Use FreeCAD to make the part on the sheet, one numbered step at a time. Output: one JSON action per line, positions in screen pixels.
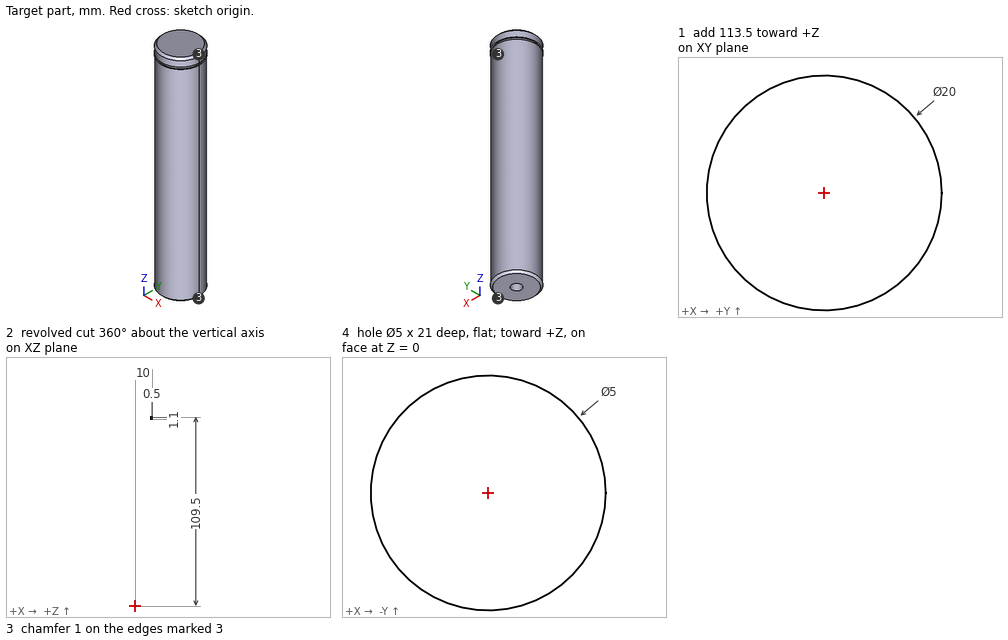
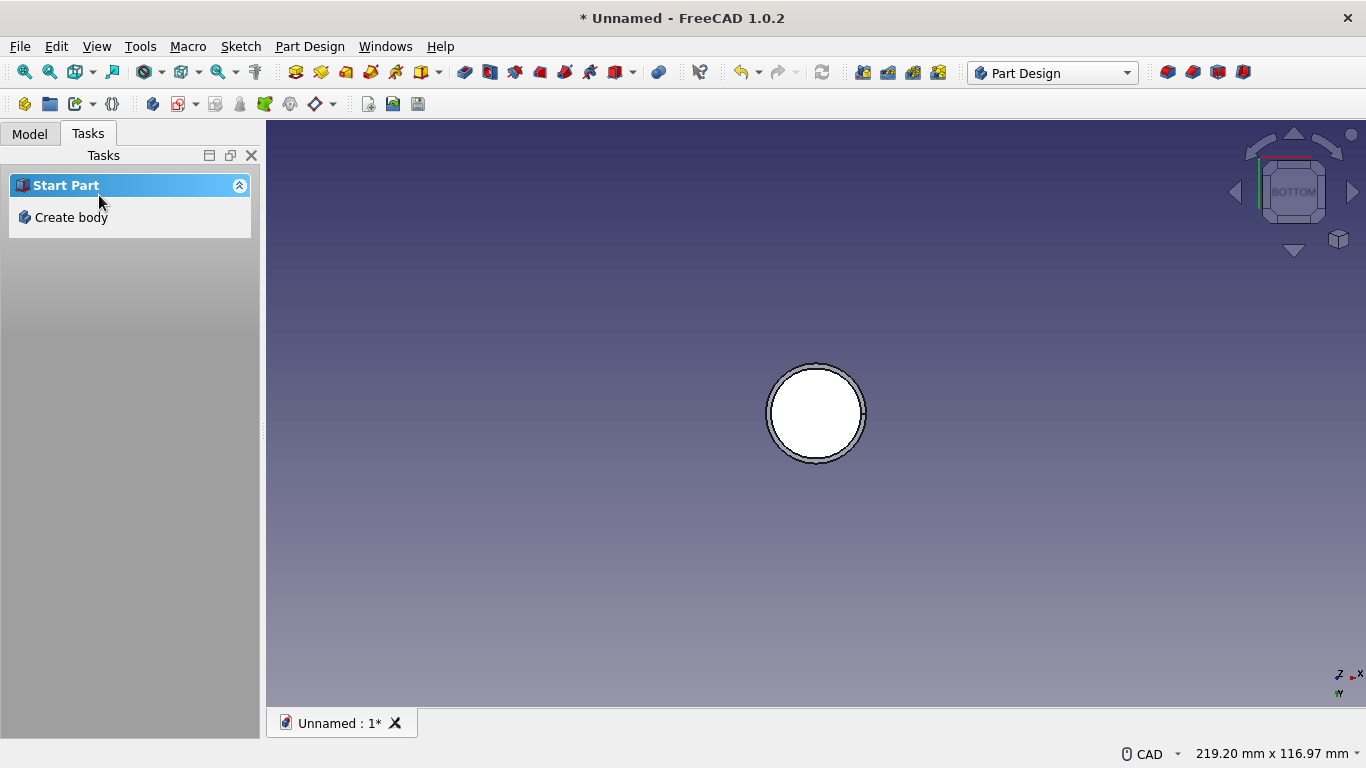
{"action": "left_click", "coordinate": [816, 412]}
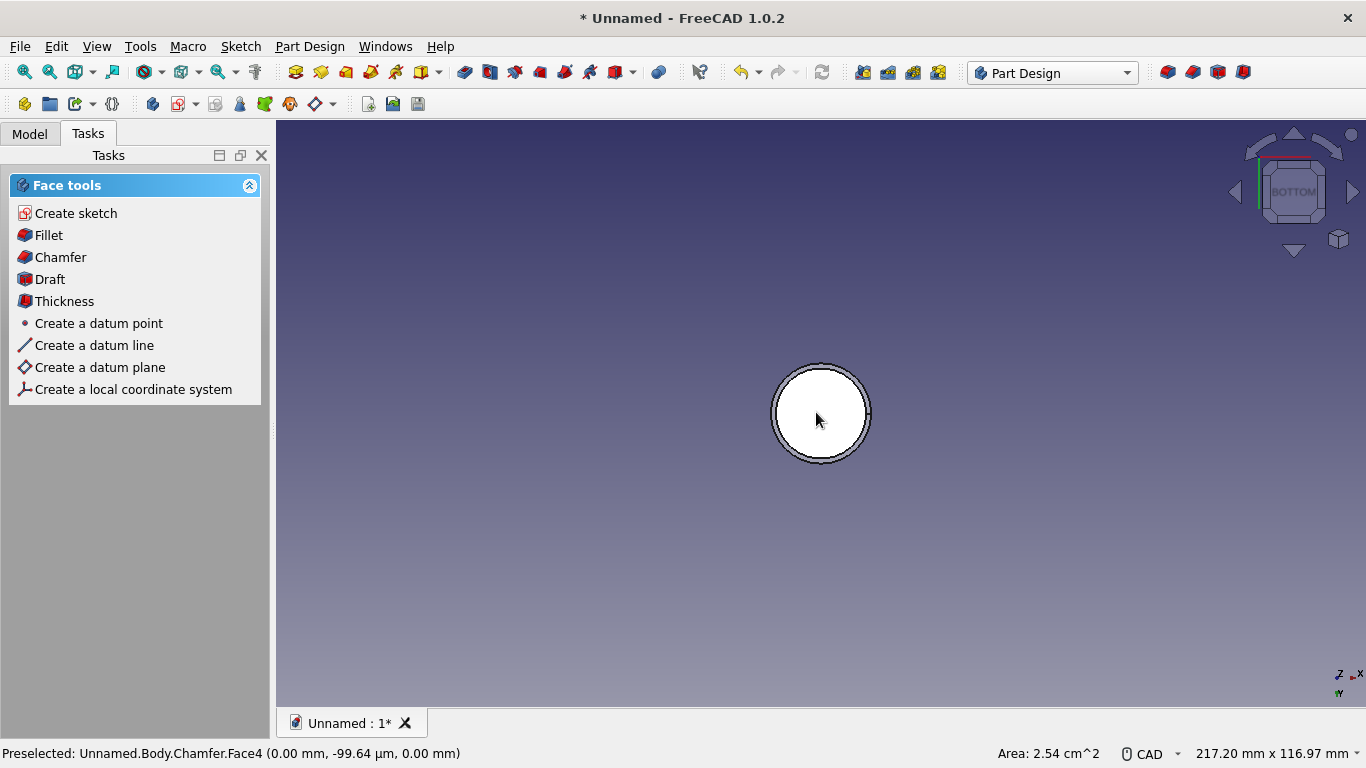
{"action": "left_click", "coordinate": [178, 104]}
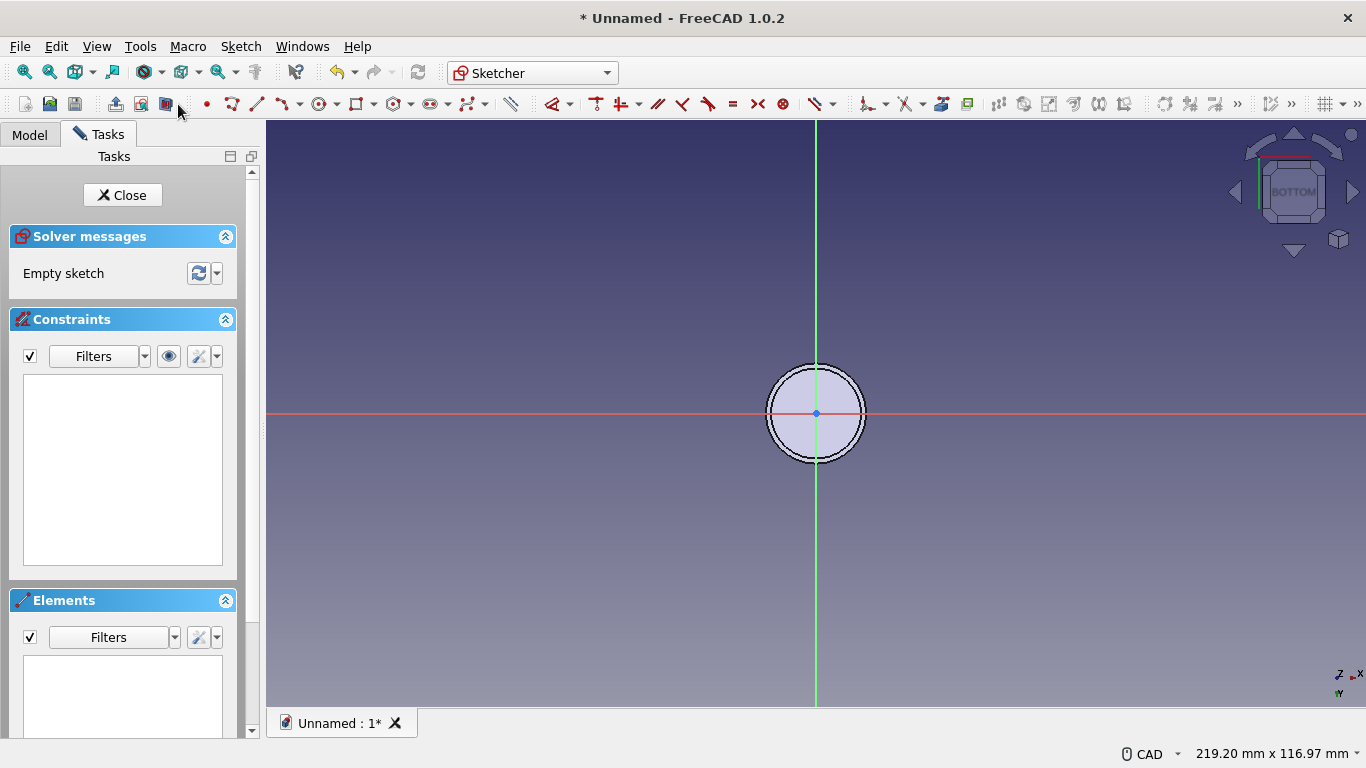
{"action": "scroll", "coordinate": [820, 414], "scroll_direction": "up", "scroll_amount": 14}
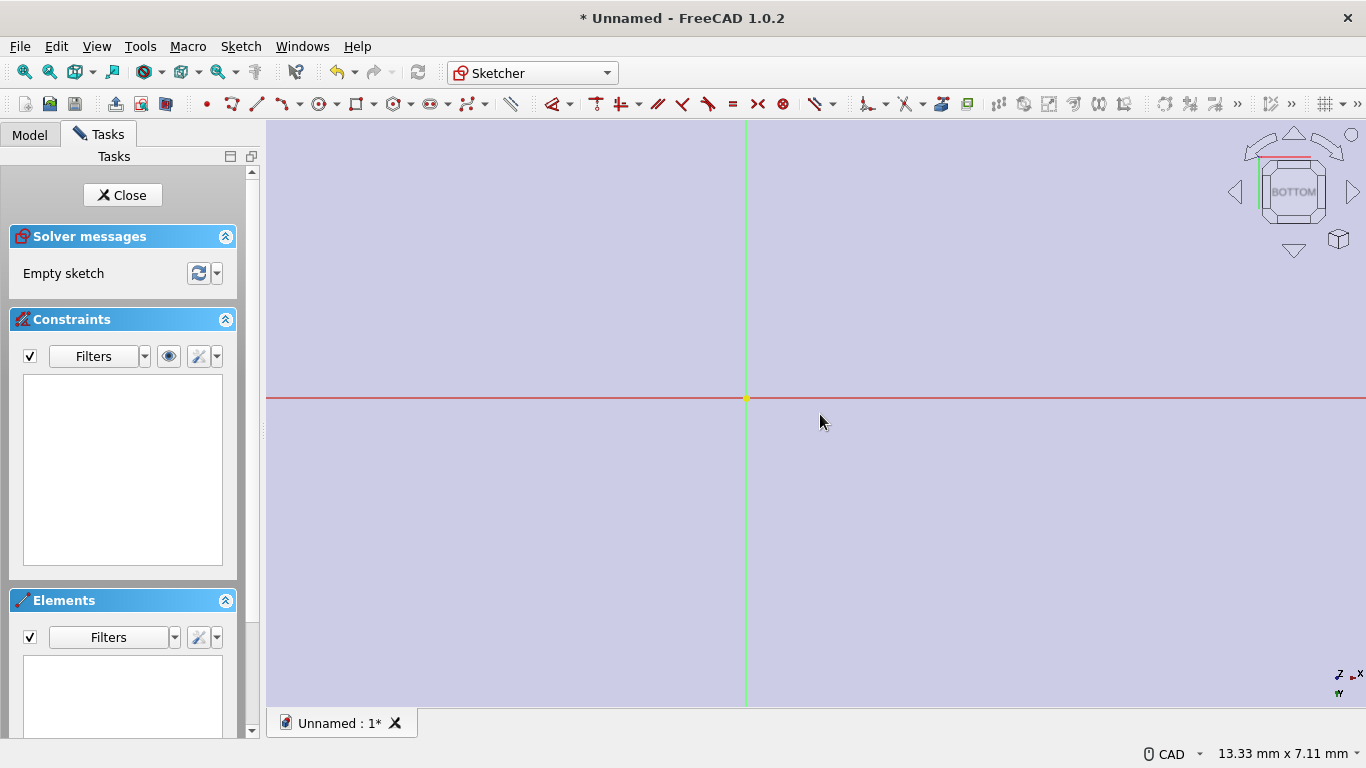
{"action": "left_click", "coordinate": [318, 104]}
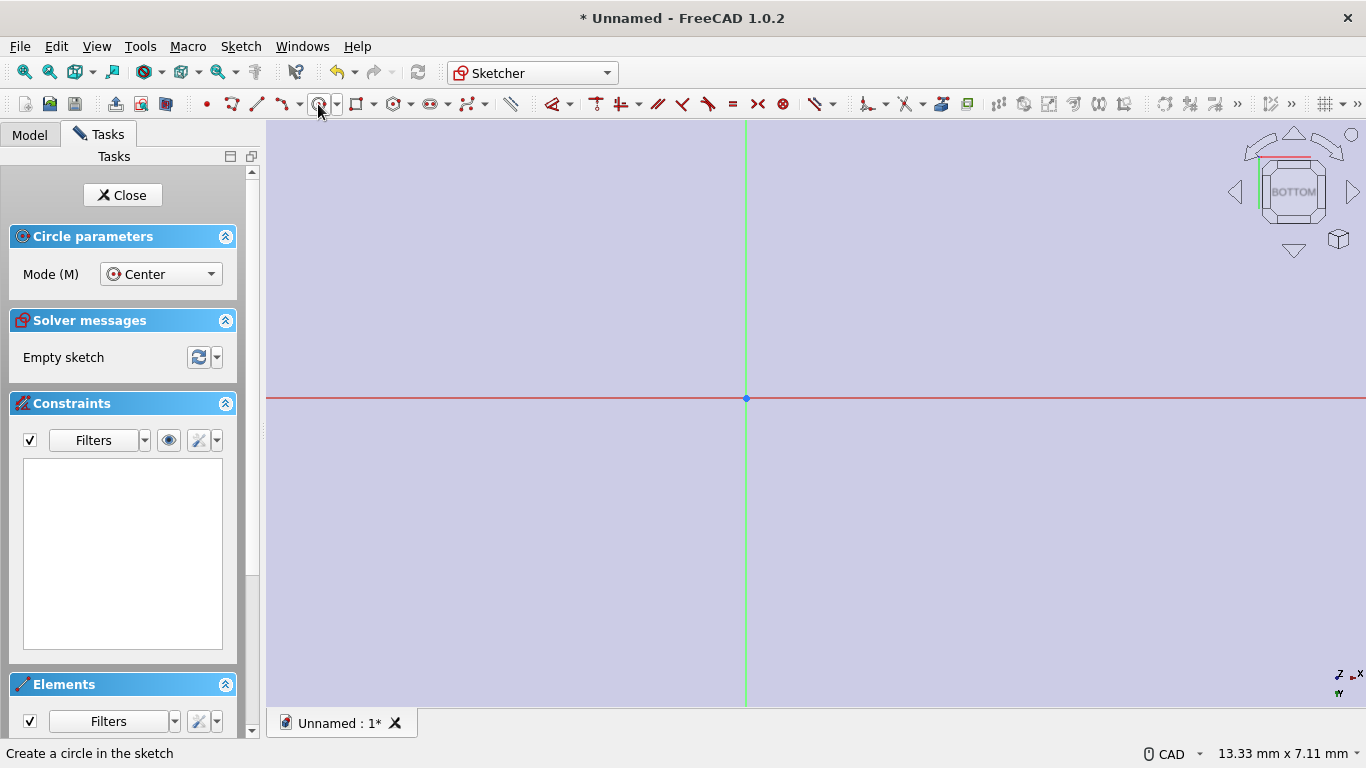
{"action": "left_click", "coordinate": [746, 398]}
{"action": "left_click", "coordinate": [892, 252]}
{"action": "key", "text": "Escape"}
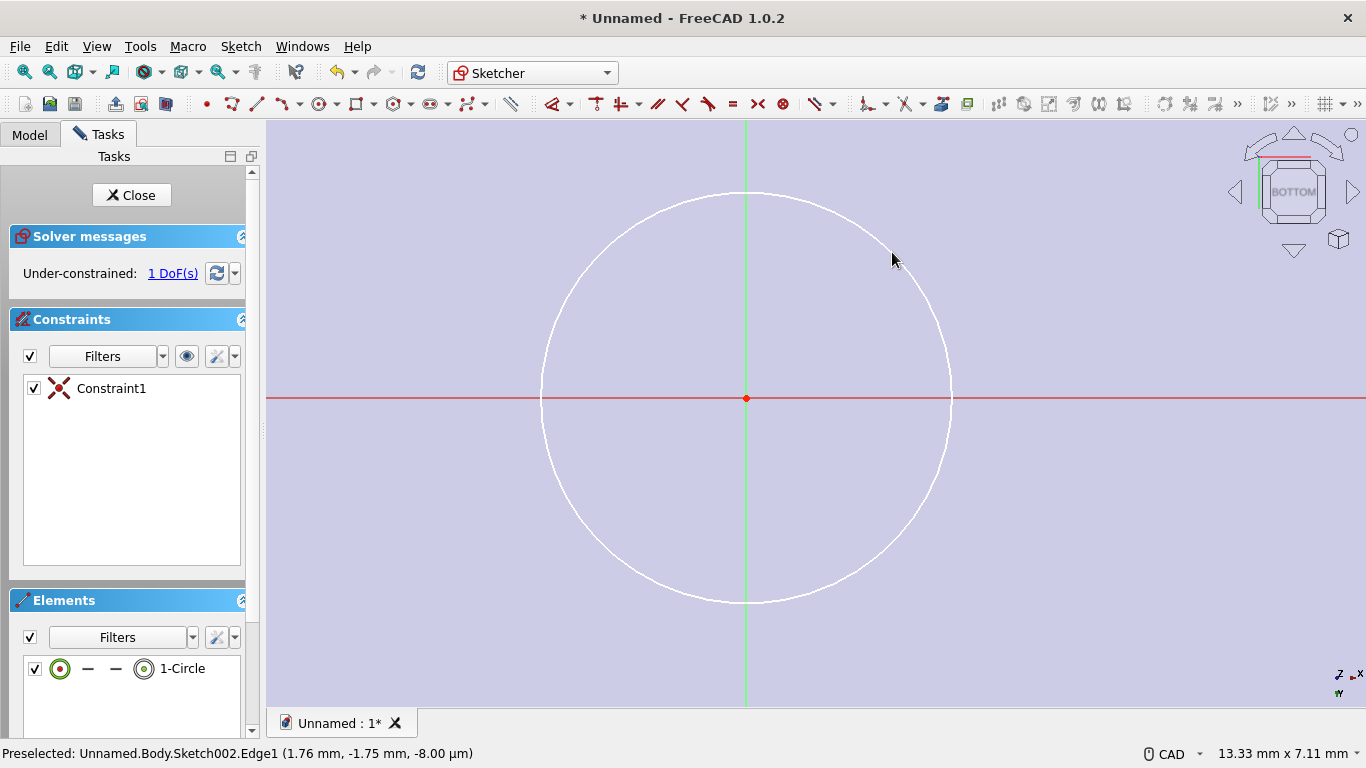
{"action": "key", "text": "d"}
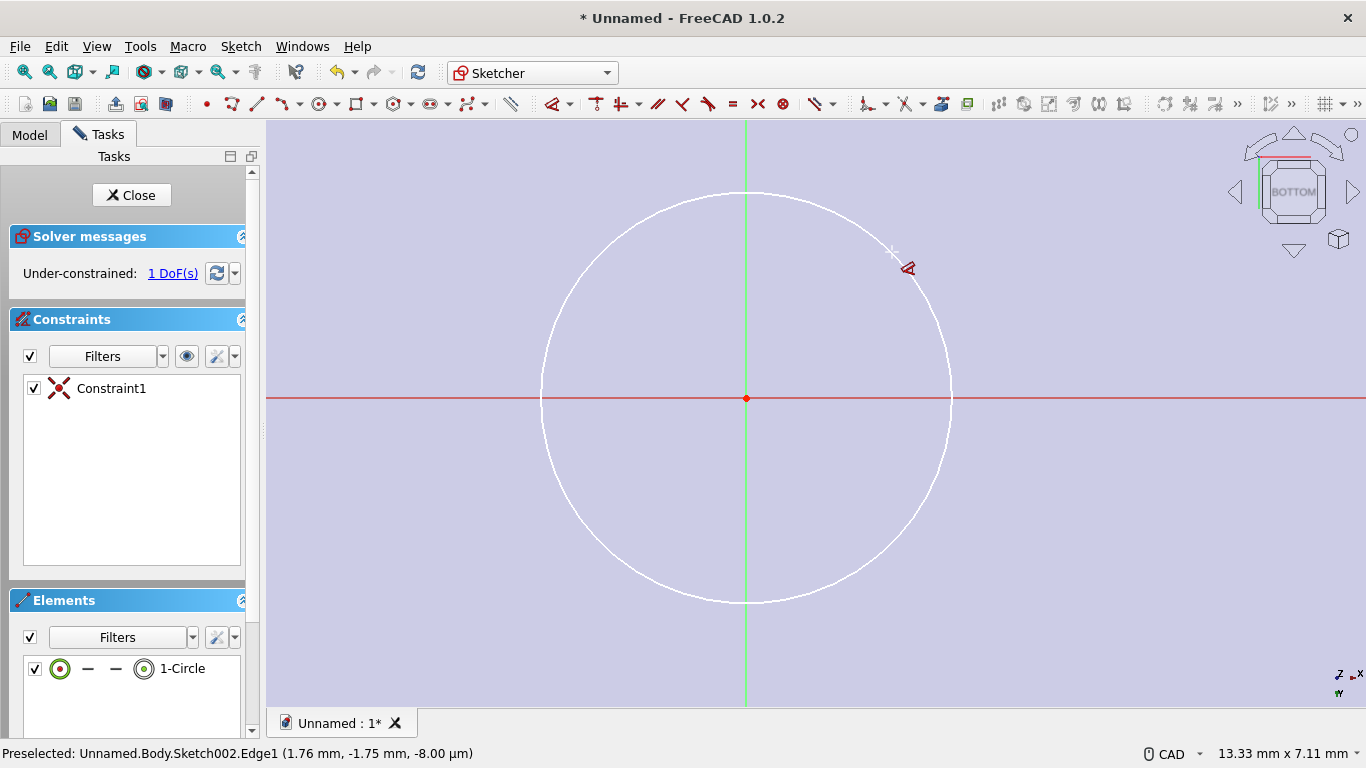
{"action": "left_click", "coordinate": [891, 252]}
{"action": "left_click", "coordinate": [914, 229]}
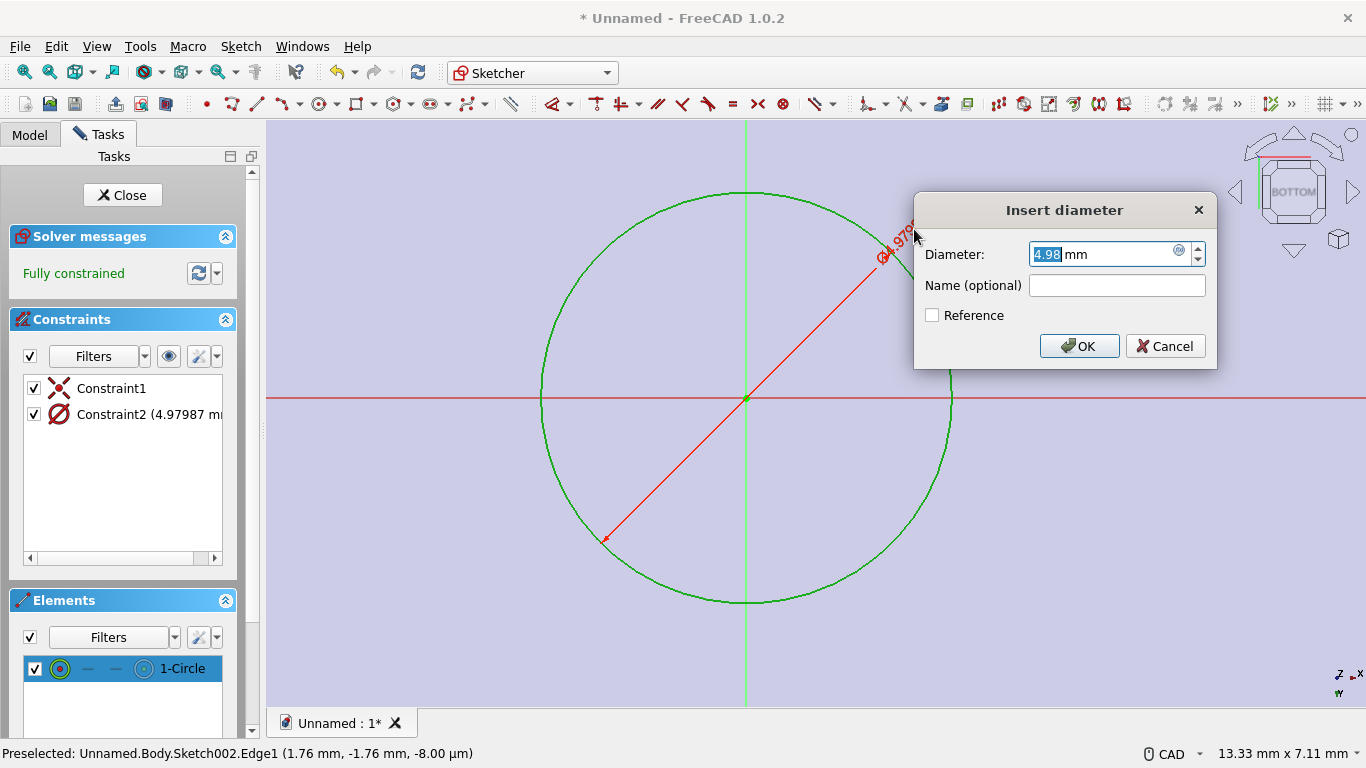
{"action": "type", "text": "5"}
{"action": "key", "text": "Return"}
{"action": "key", "text": "Escape"}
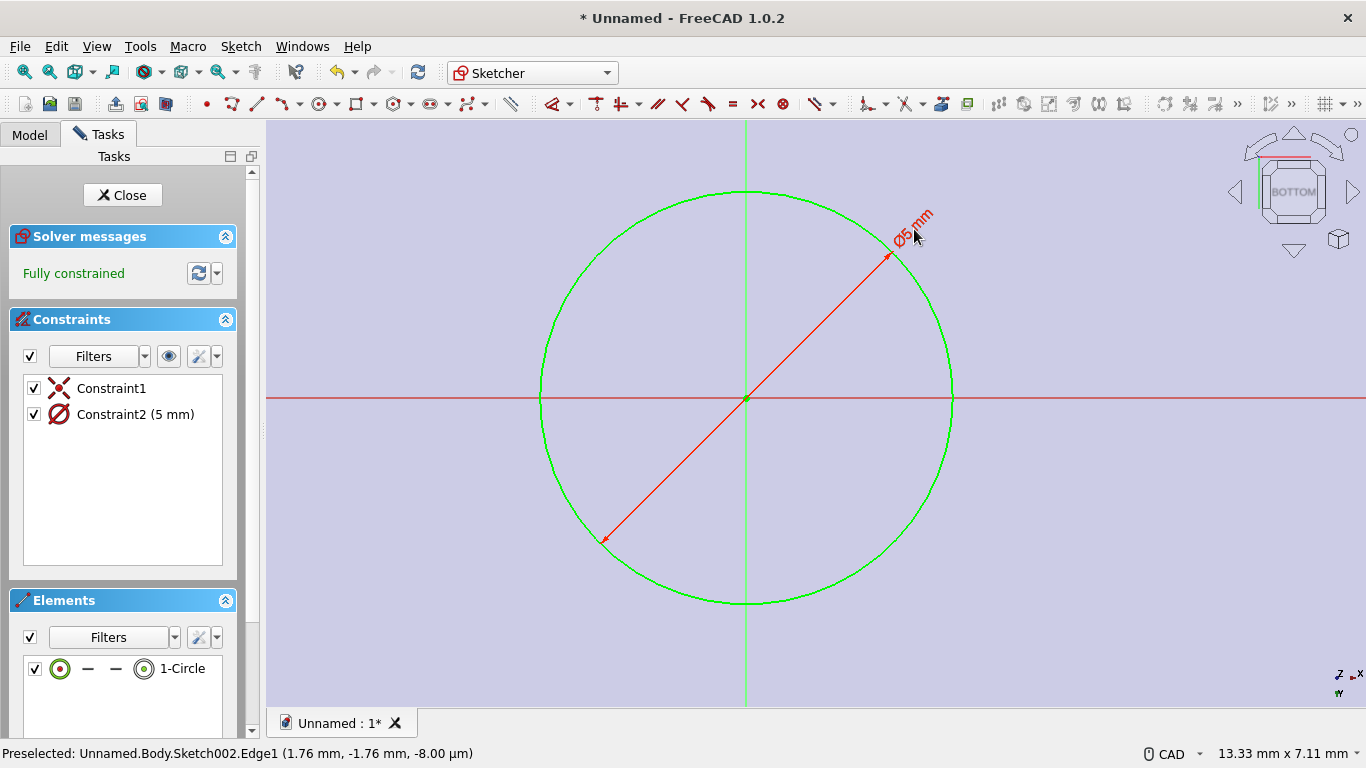
{"action": "left_click", "coordinate": [123, 195]}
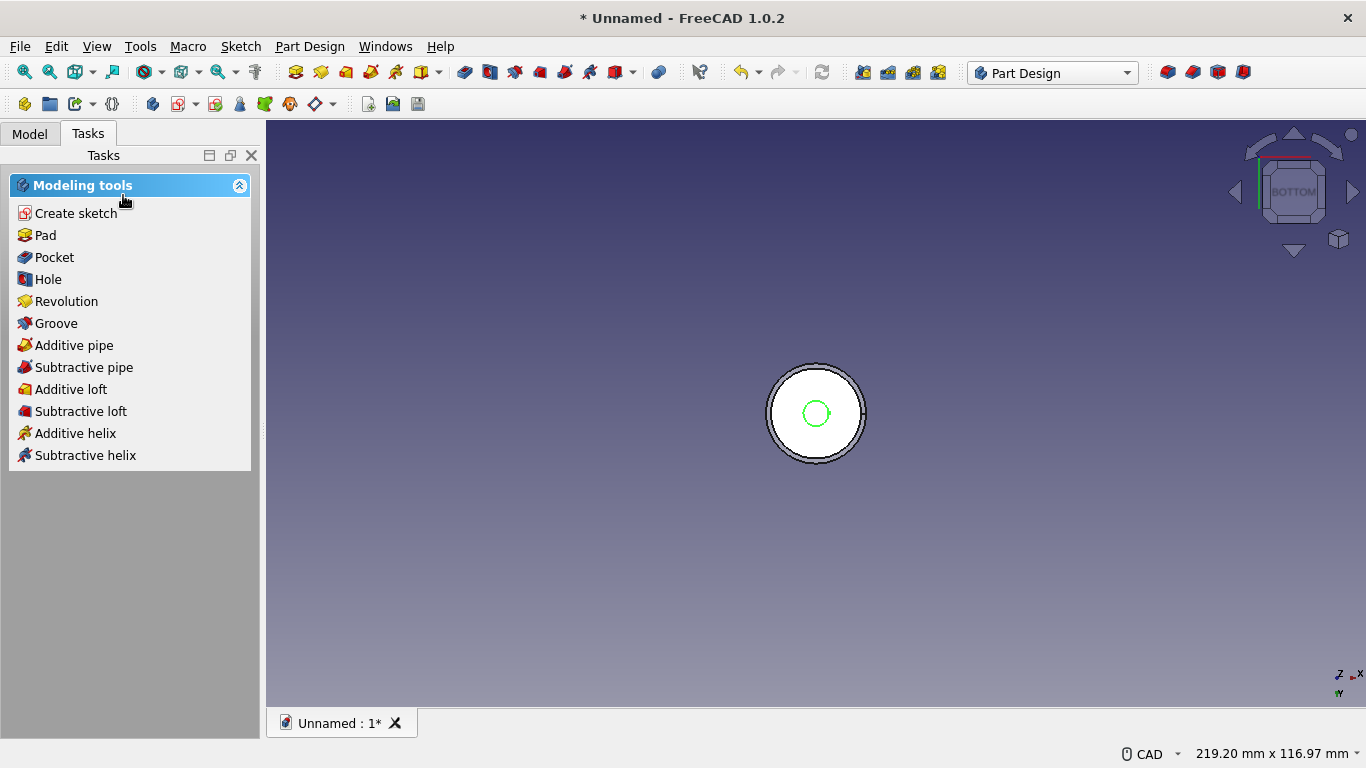
{"action": "left_click", "coordinate": [490, 72]}